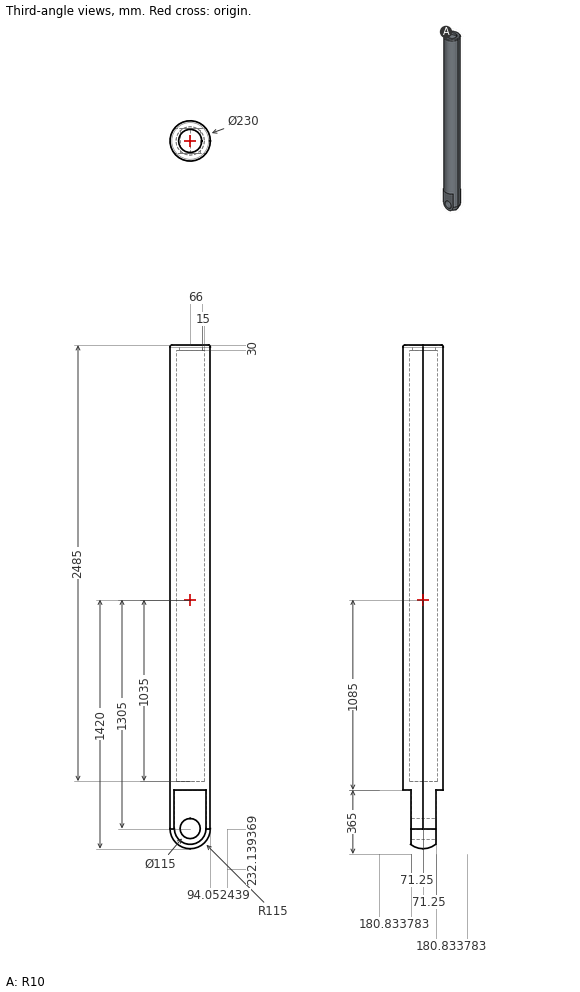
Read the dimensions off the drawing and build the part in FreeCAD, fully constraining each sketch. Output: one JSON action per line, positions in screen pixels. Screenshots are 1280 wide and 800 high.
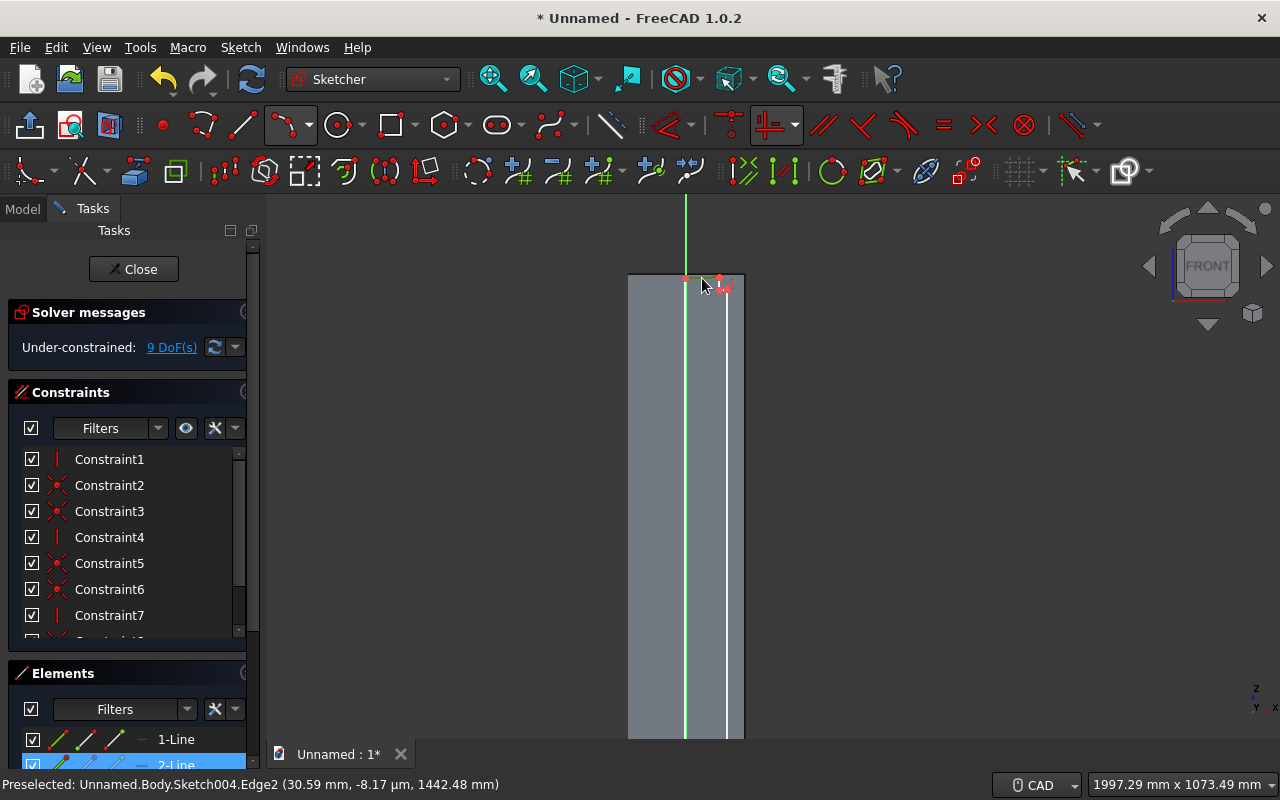
{"action": "key", "text": "h"}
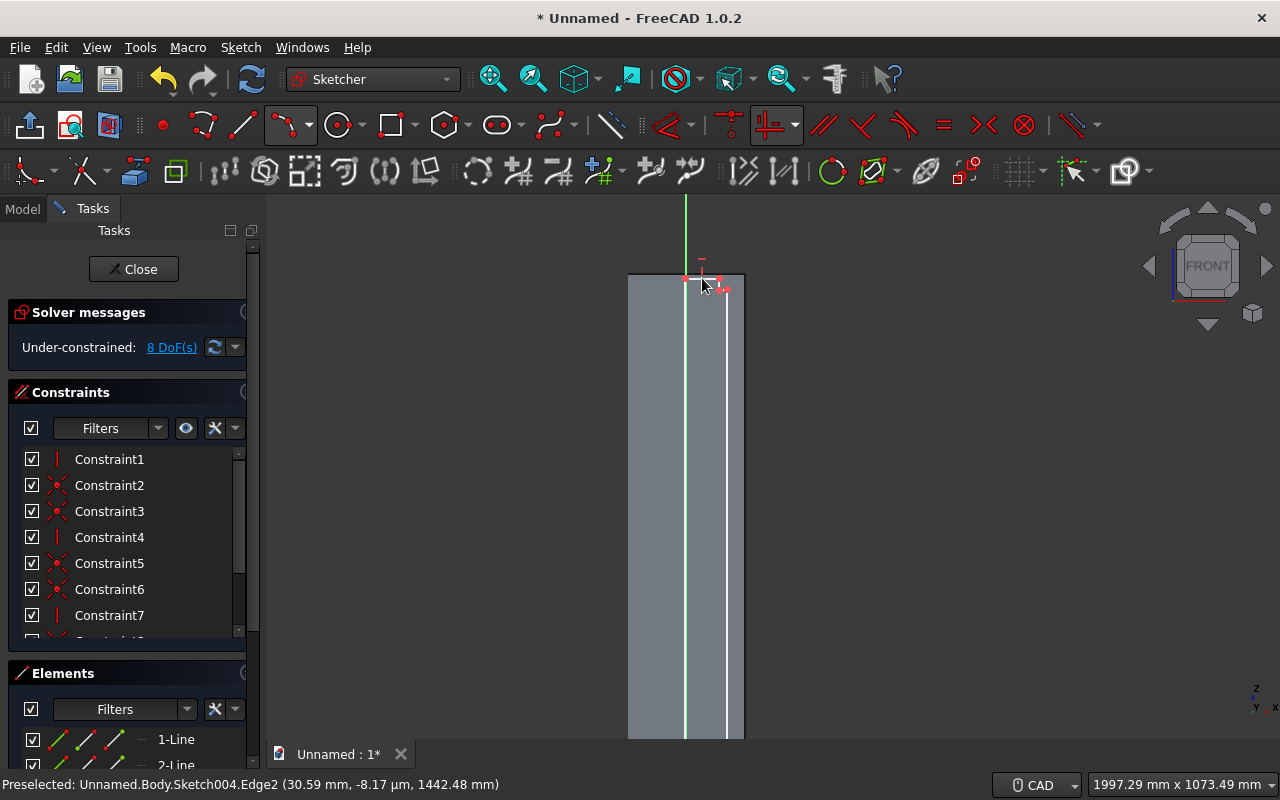
{"action": "scroll", "coordinate": [723, 290], "scroll_direction": "up", "scroll_amount": 6}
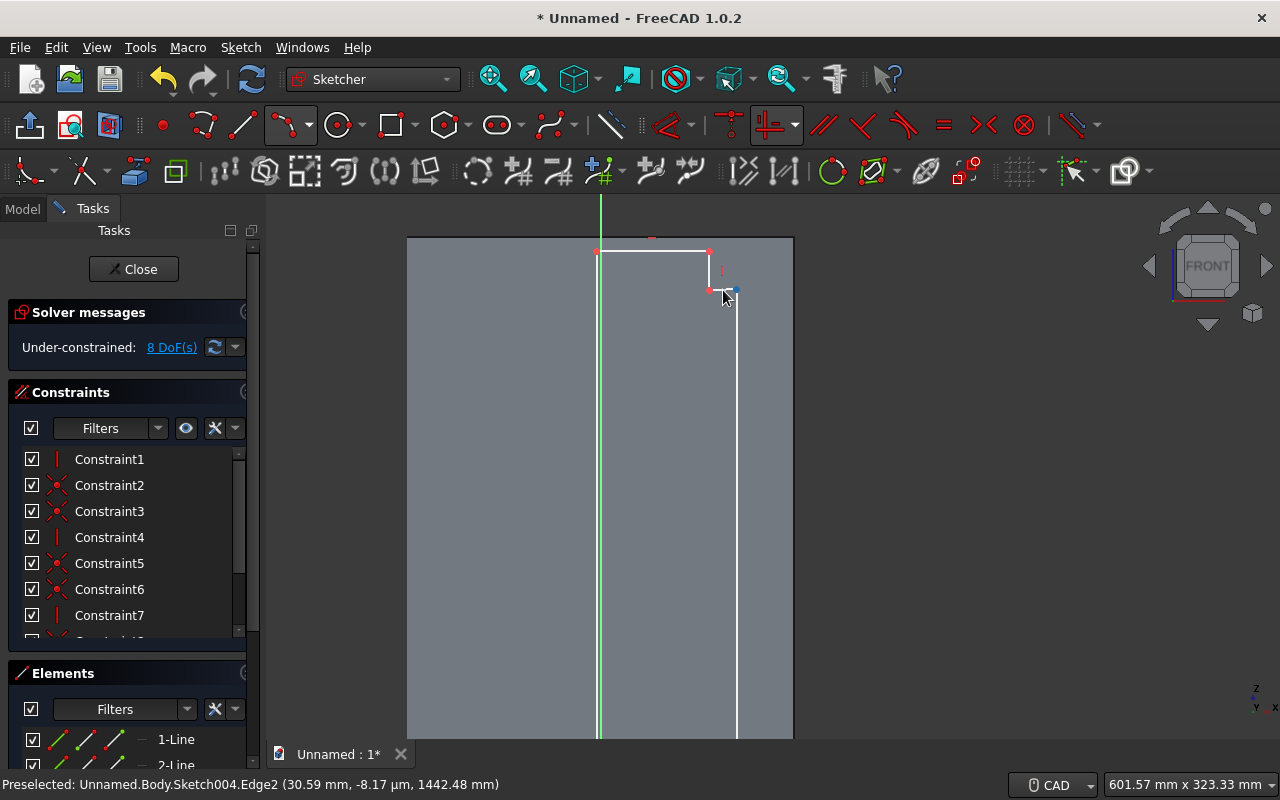
{"action": "left_click", "coordinate": [723, 290]}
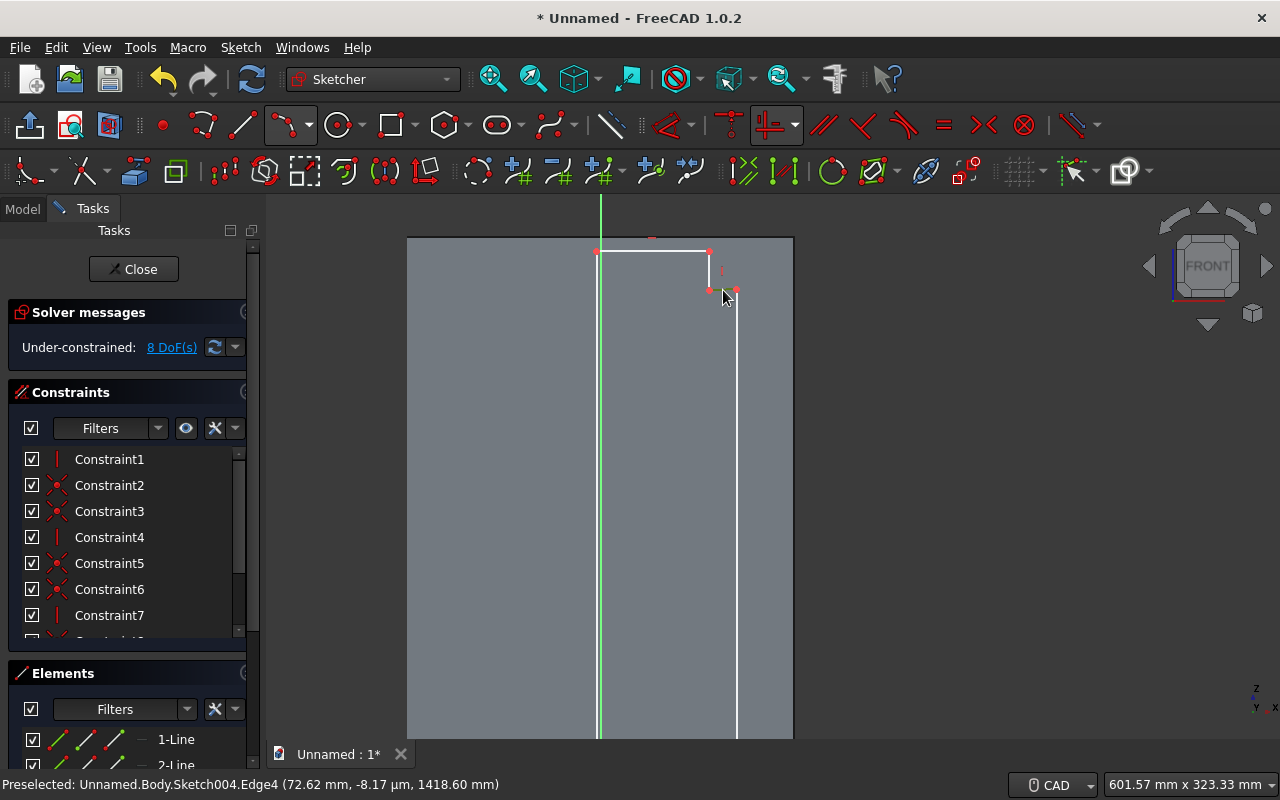
{"action": "left_click", "coordinate": [798, 126]}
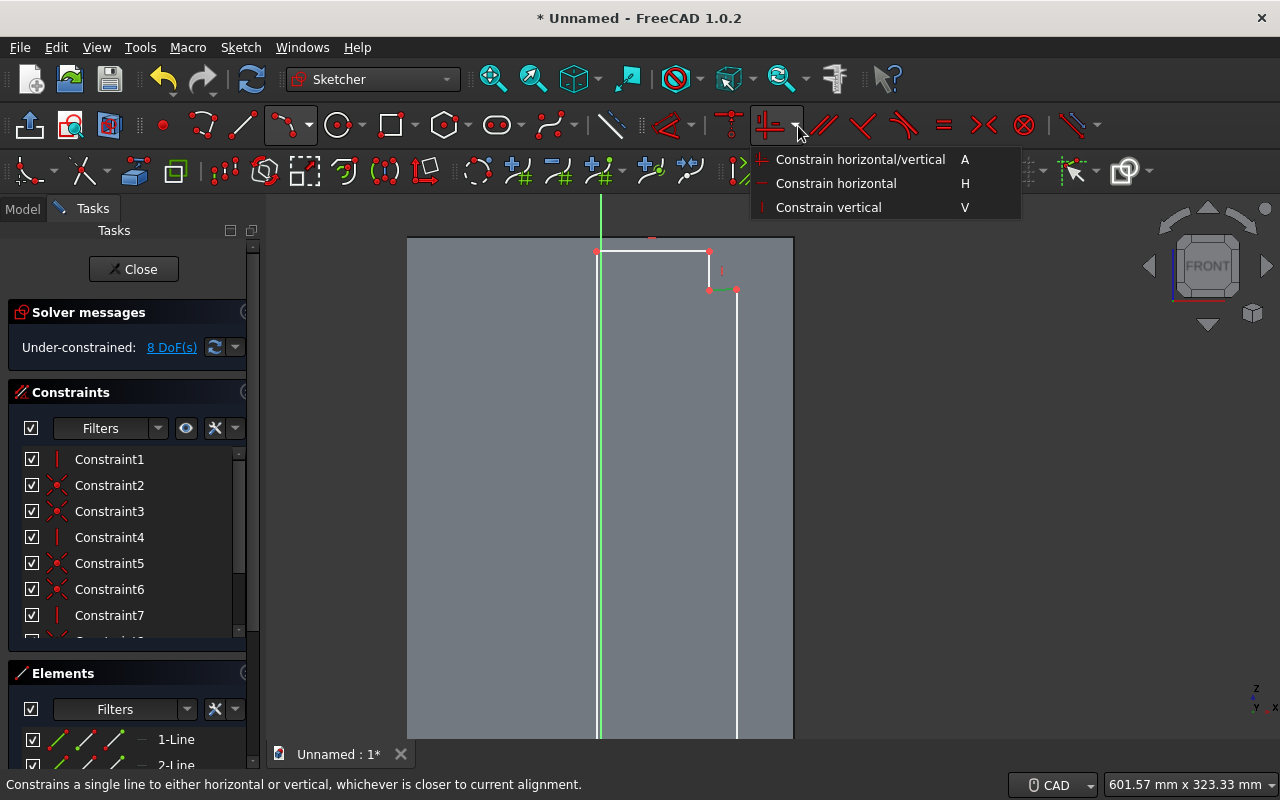
{"action": "left_click", "coordinate": [886, 183]}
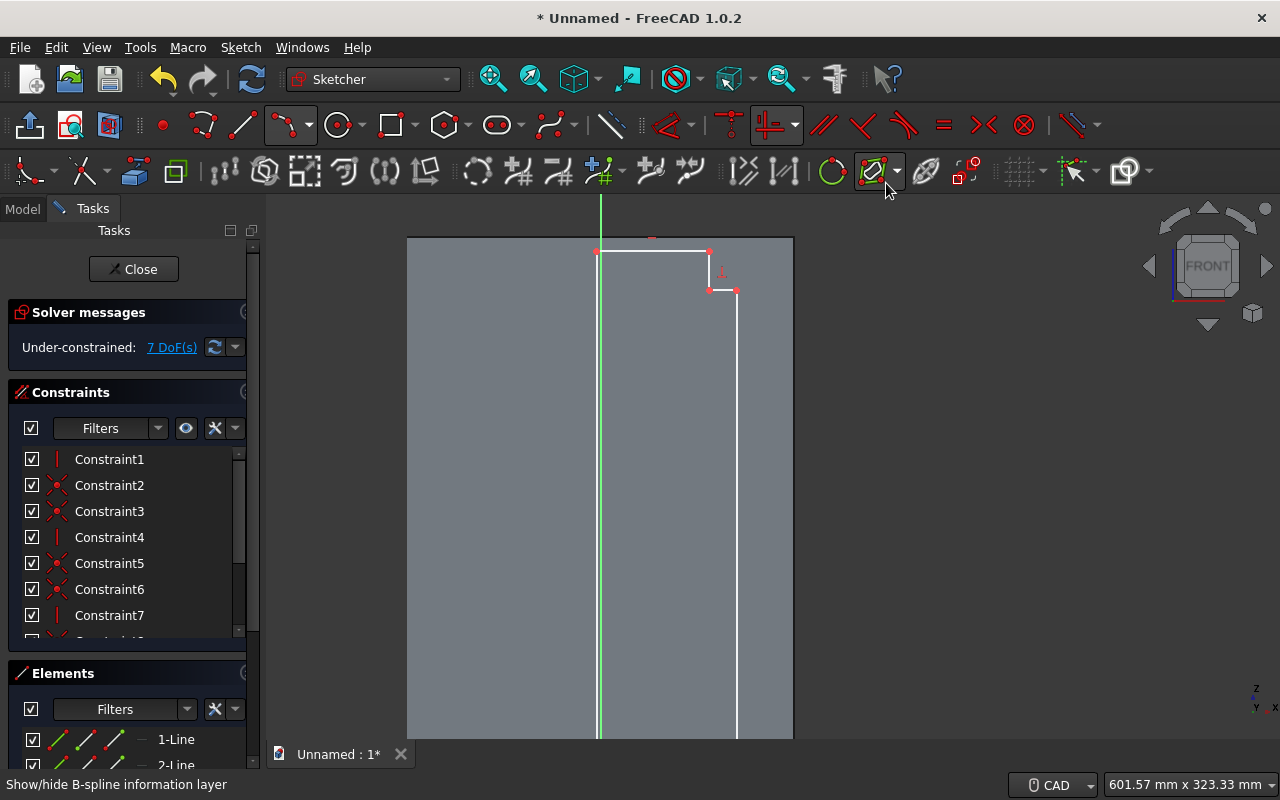
{"action": "scroll", "coordinate": [708, 280], "scroll_direction": "down", "scroll_amount": 12}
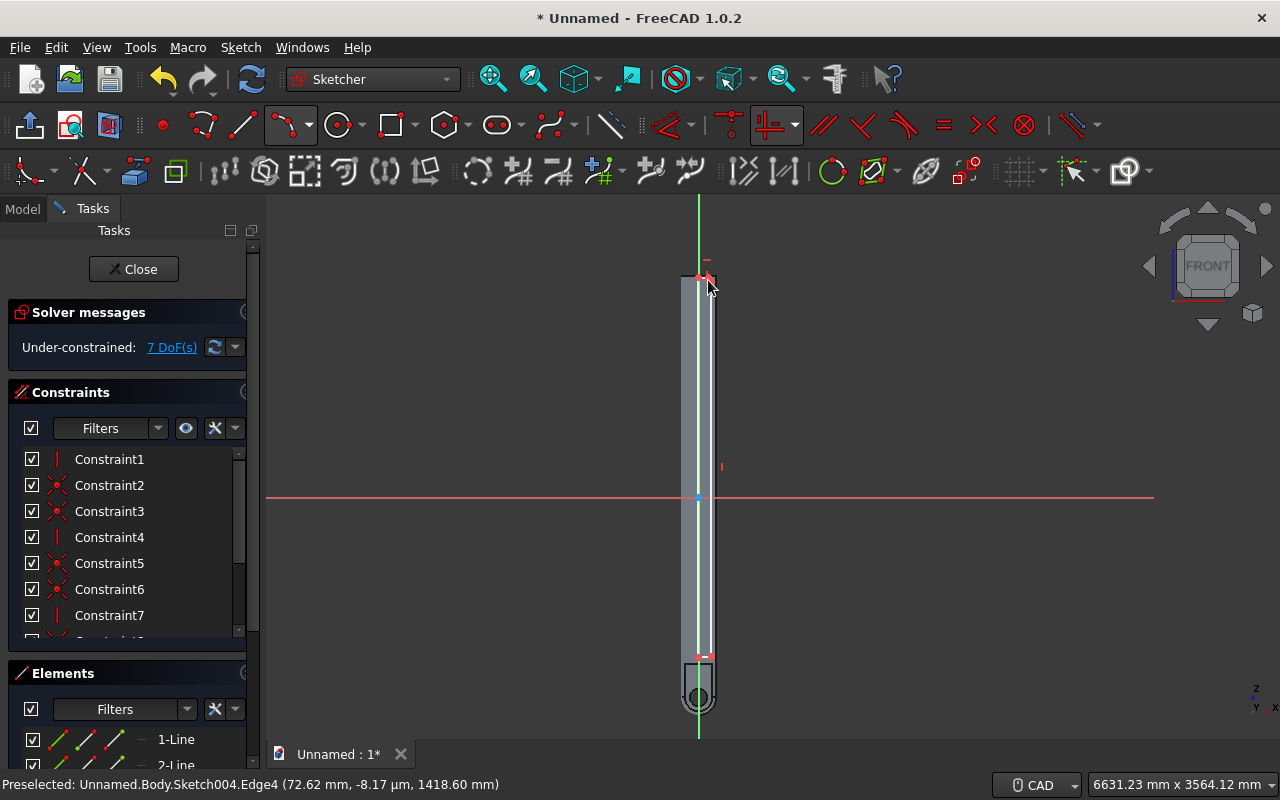
{"action": "scroll", "coordinate": [707, 657], "scroll_direction": "up", "scroll_amount": 7}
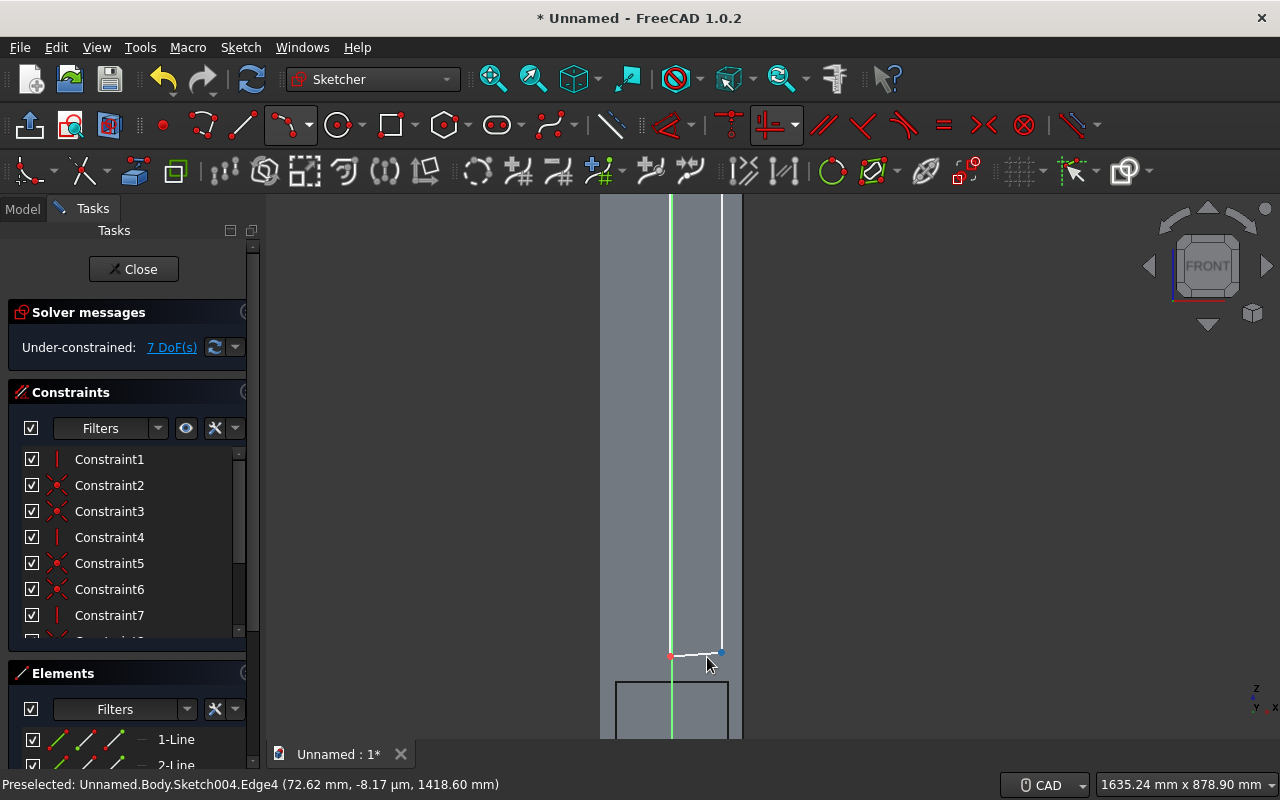
{"action": "left_click", "coordinate": [706, 654]}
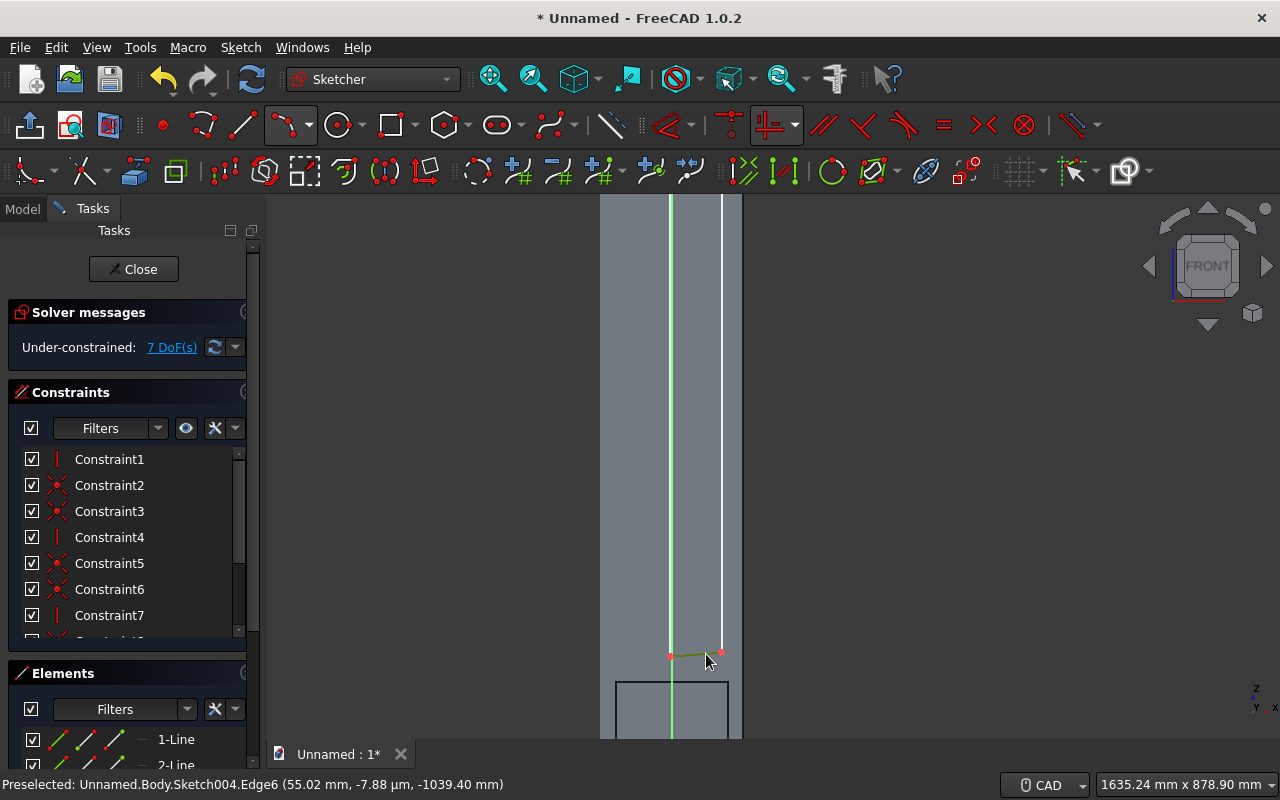
{"action": "key", "text": "h"}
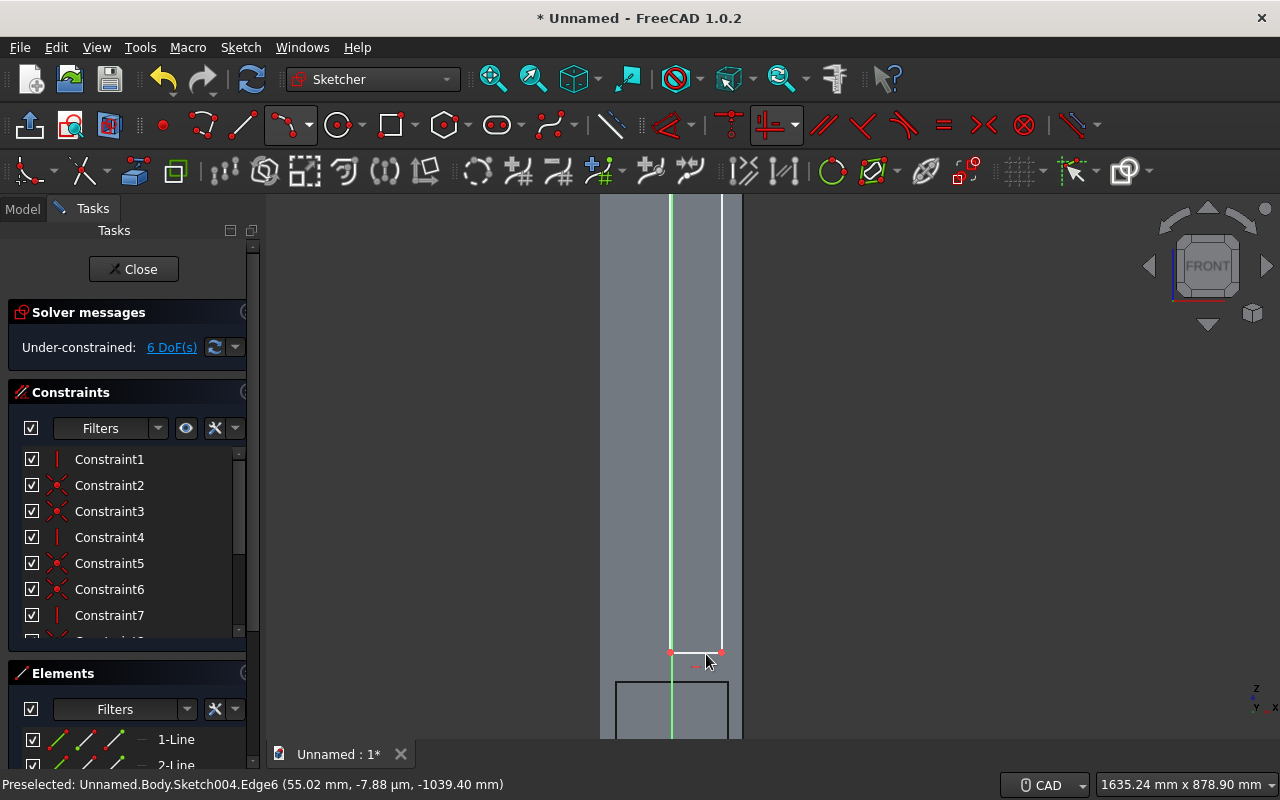
{"action": "scroll", "coordinate": [707, 658], "scroll_direction": "down", "scroll_amount": 7}